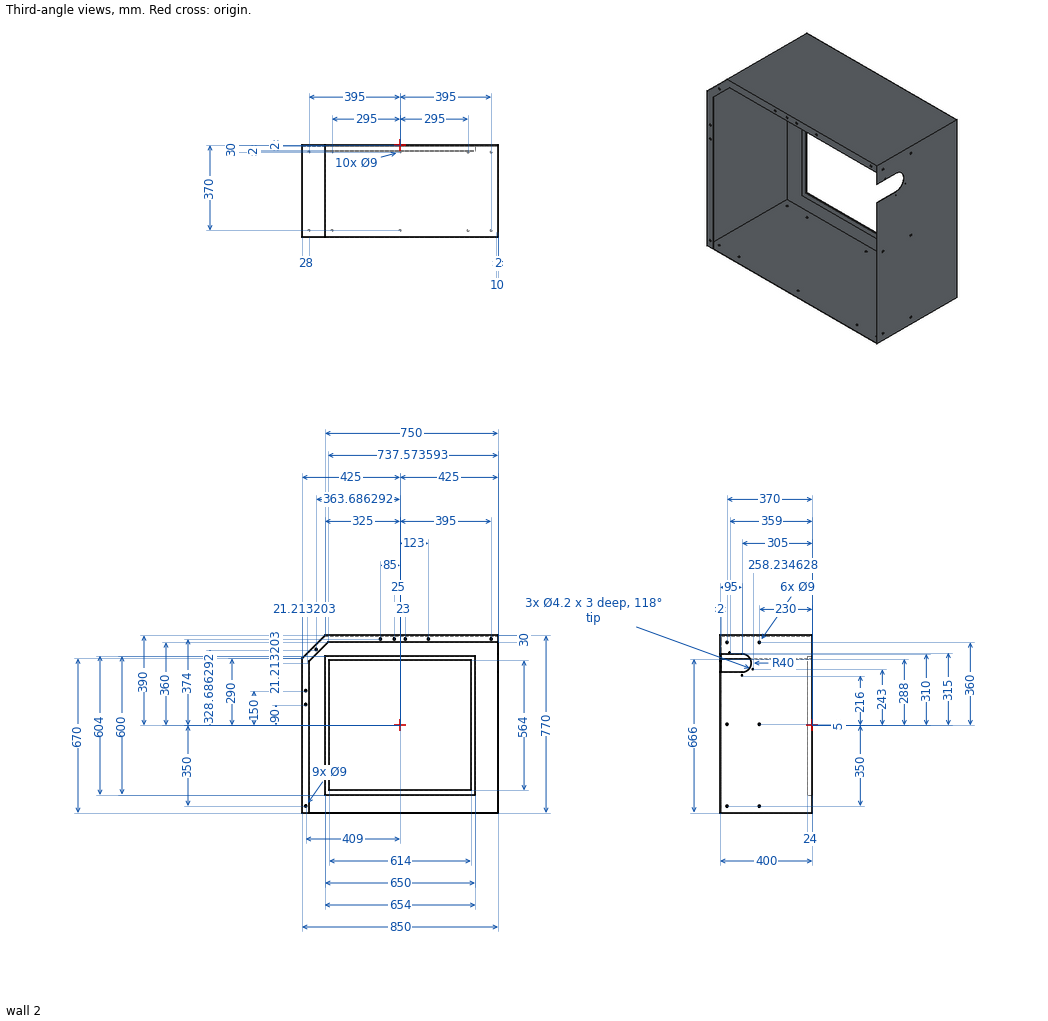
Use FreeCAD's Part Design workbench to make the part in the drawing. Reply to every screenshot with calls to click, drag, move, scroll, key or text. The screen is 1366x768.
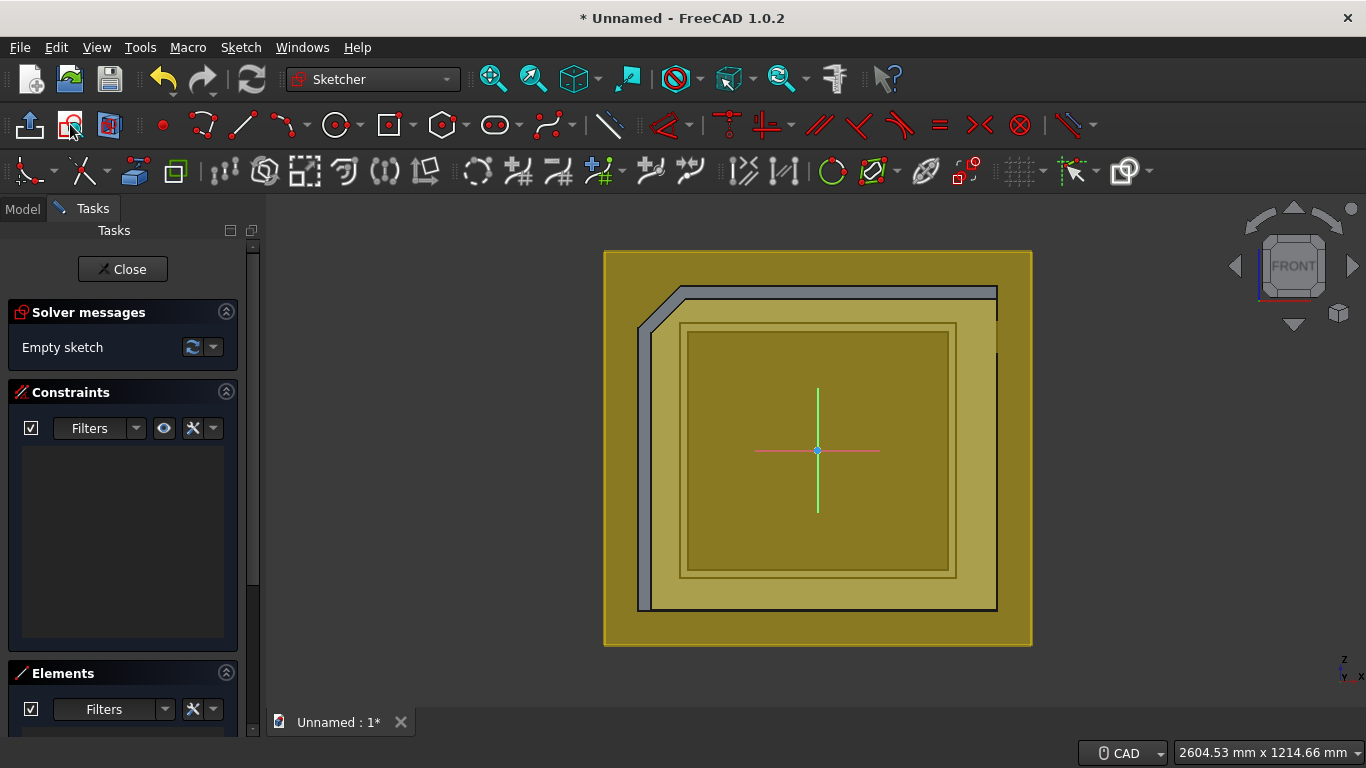
click(110, 126)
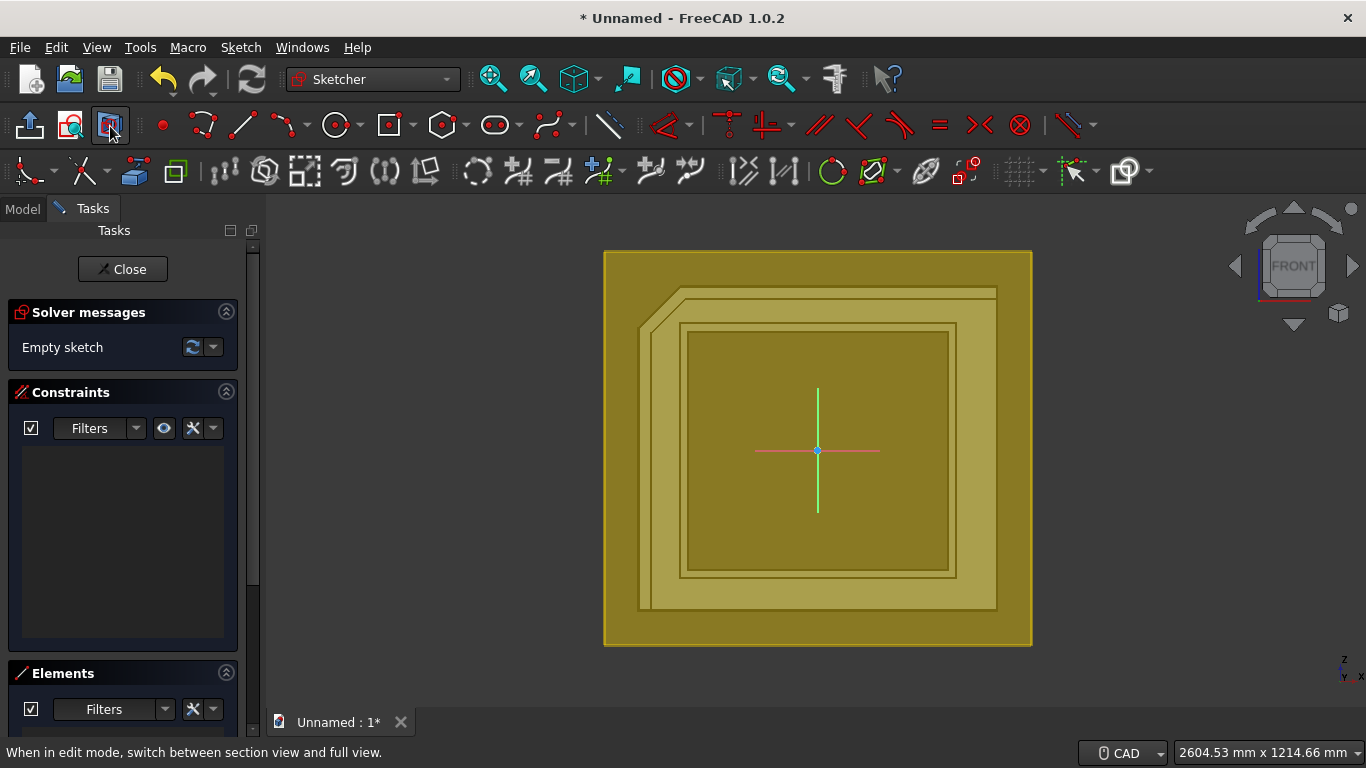
click(336, 126)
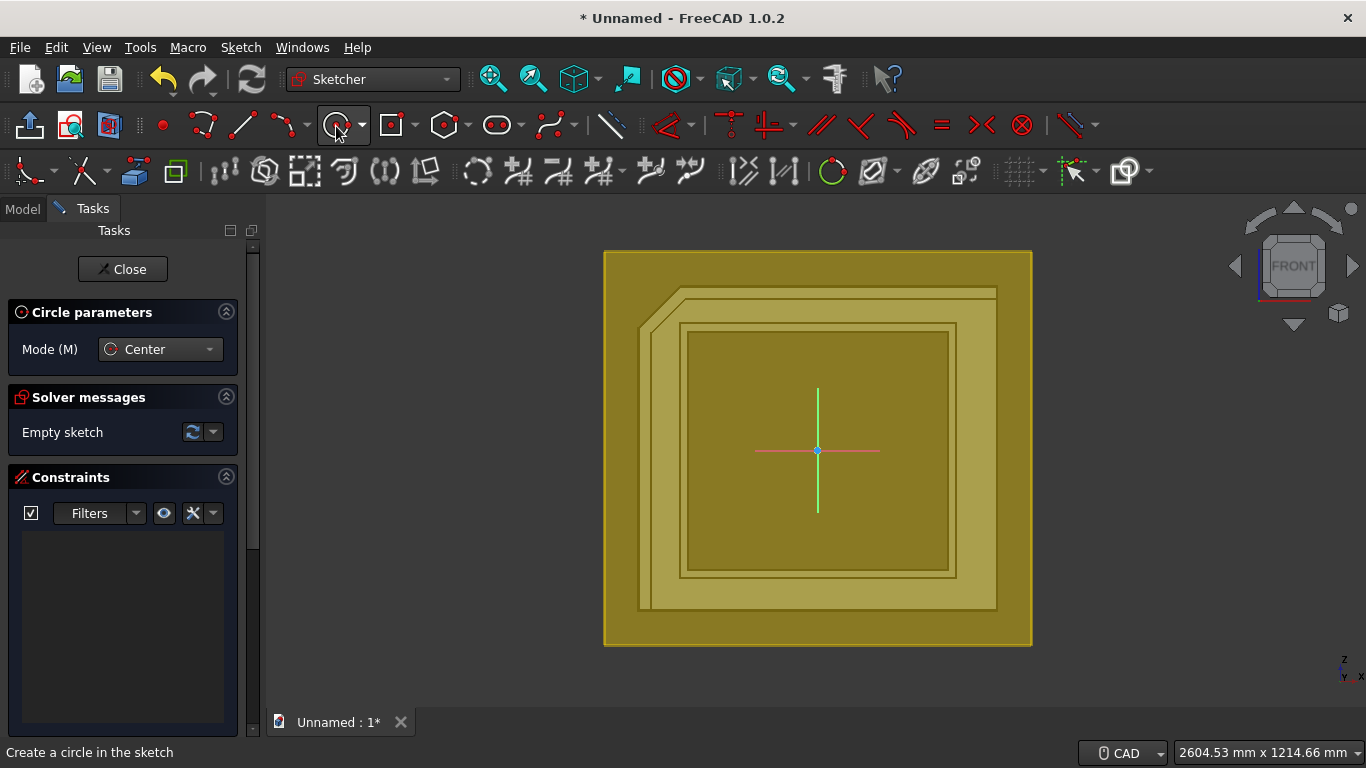
scroll(645, 598, up, 13)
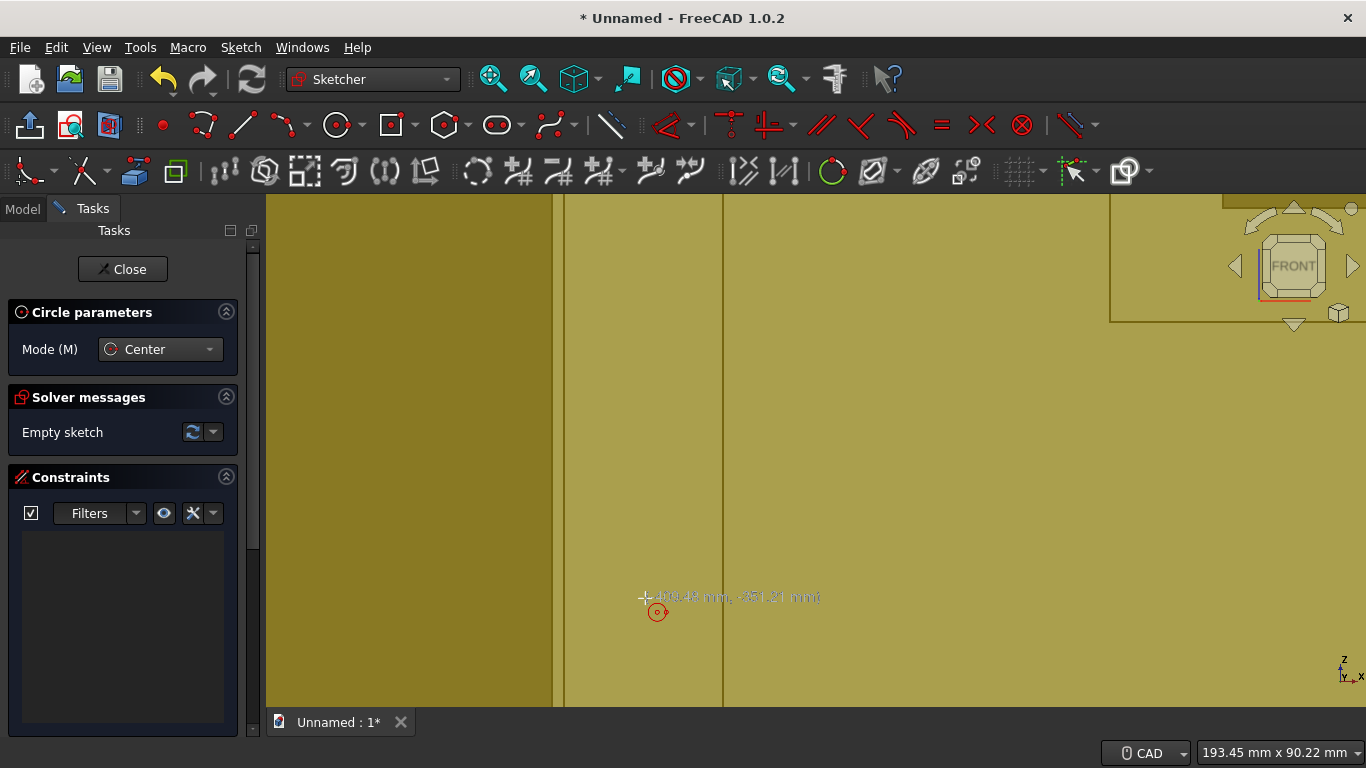
scroll(572, 604, down, 13)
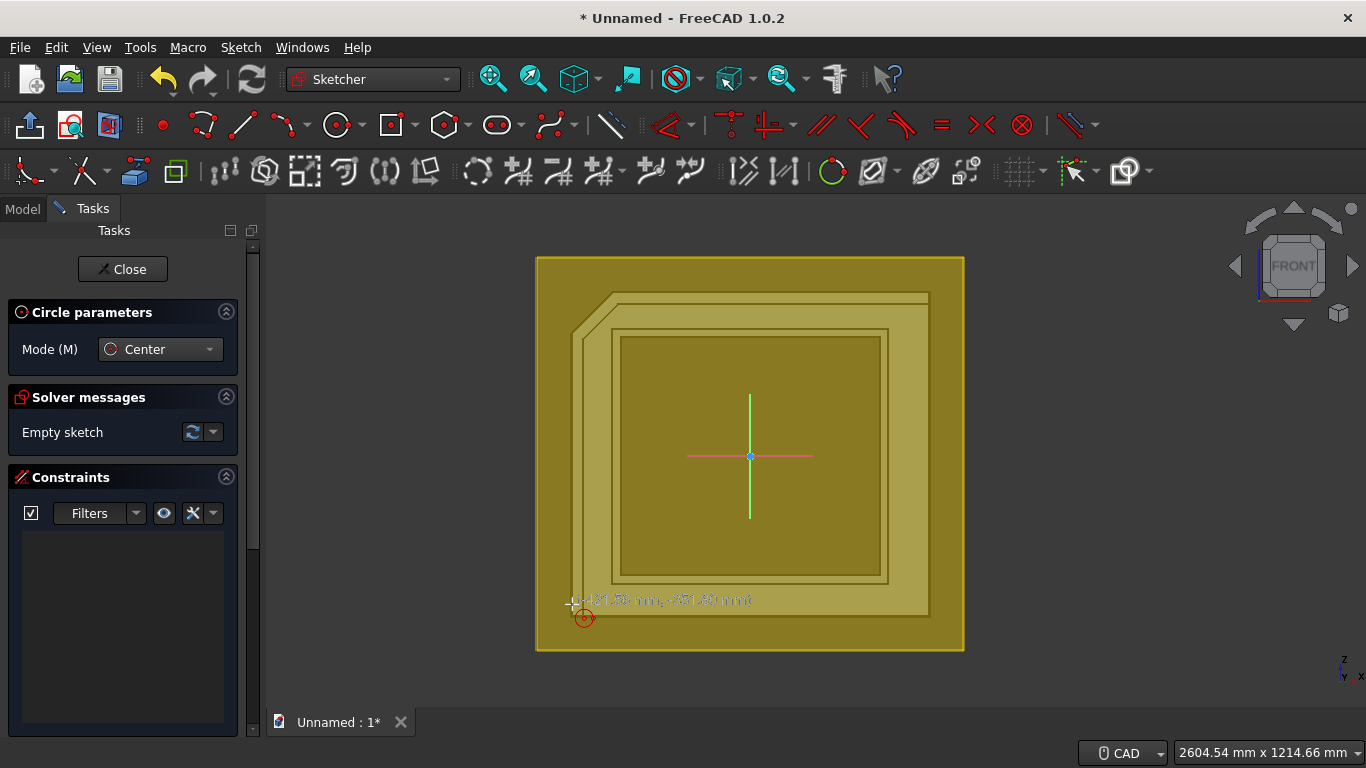
click(578, 604)
move(579, 603)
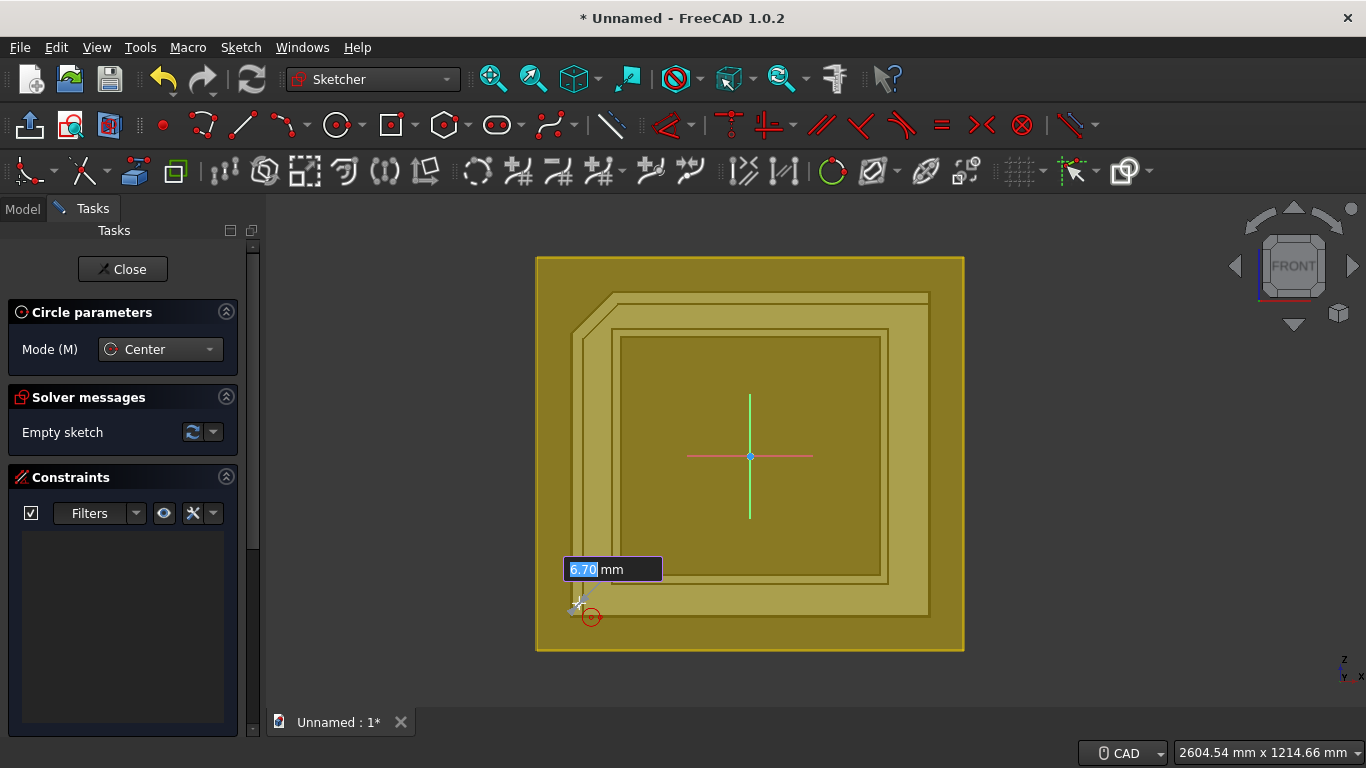
text(9)
key(Return)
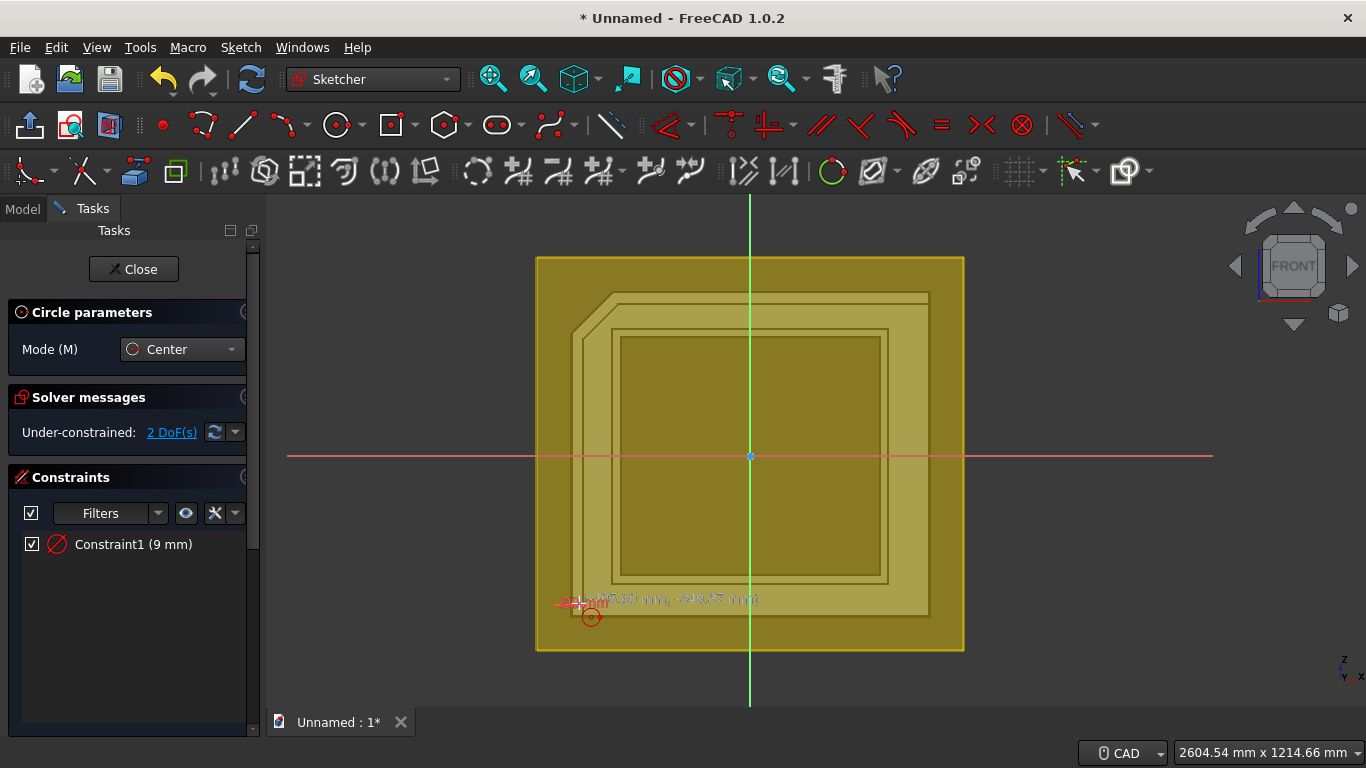
scroll(597, 317, up, 13)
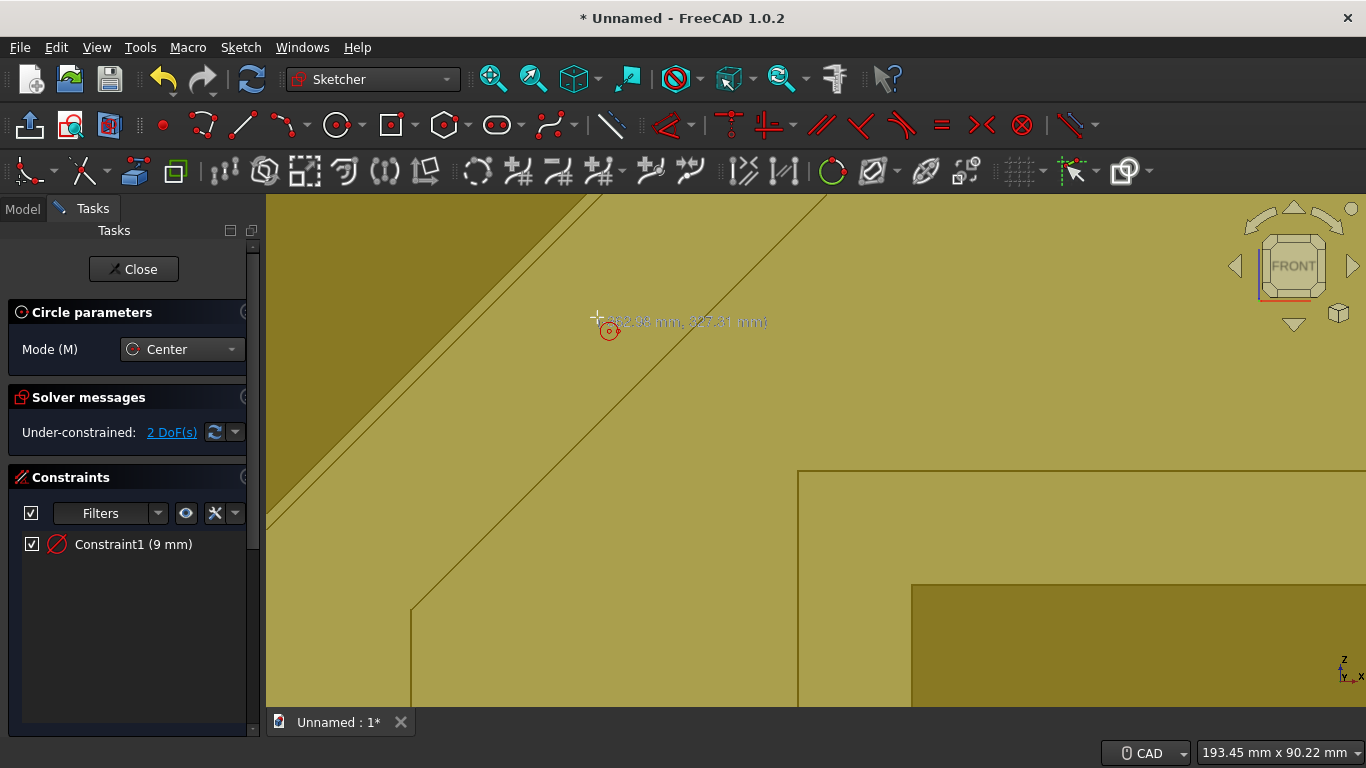
scroll(597, 317, down, 13)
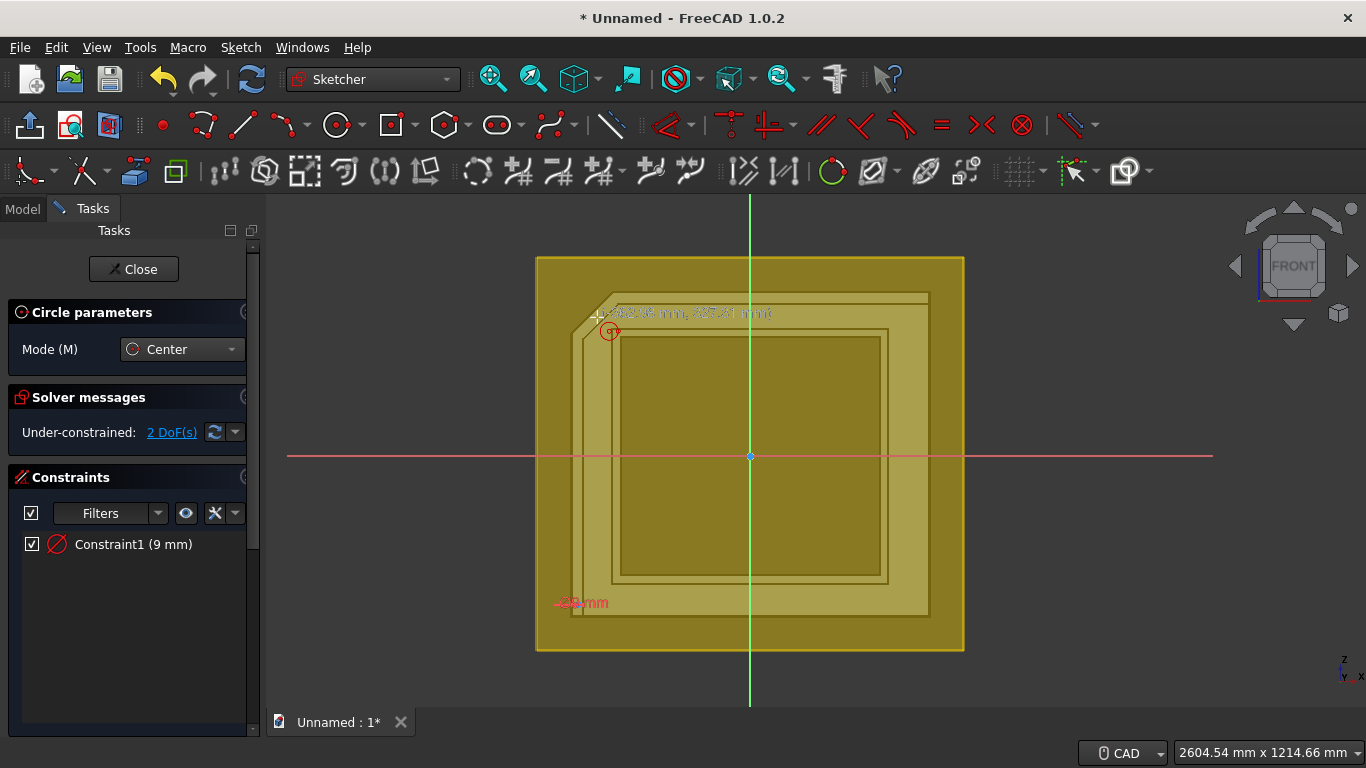
click(597, 317)
move(598, 316)